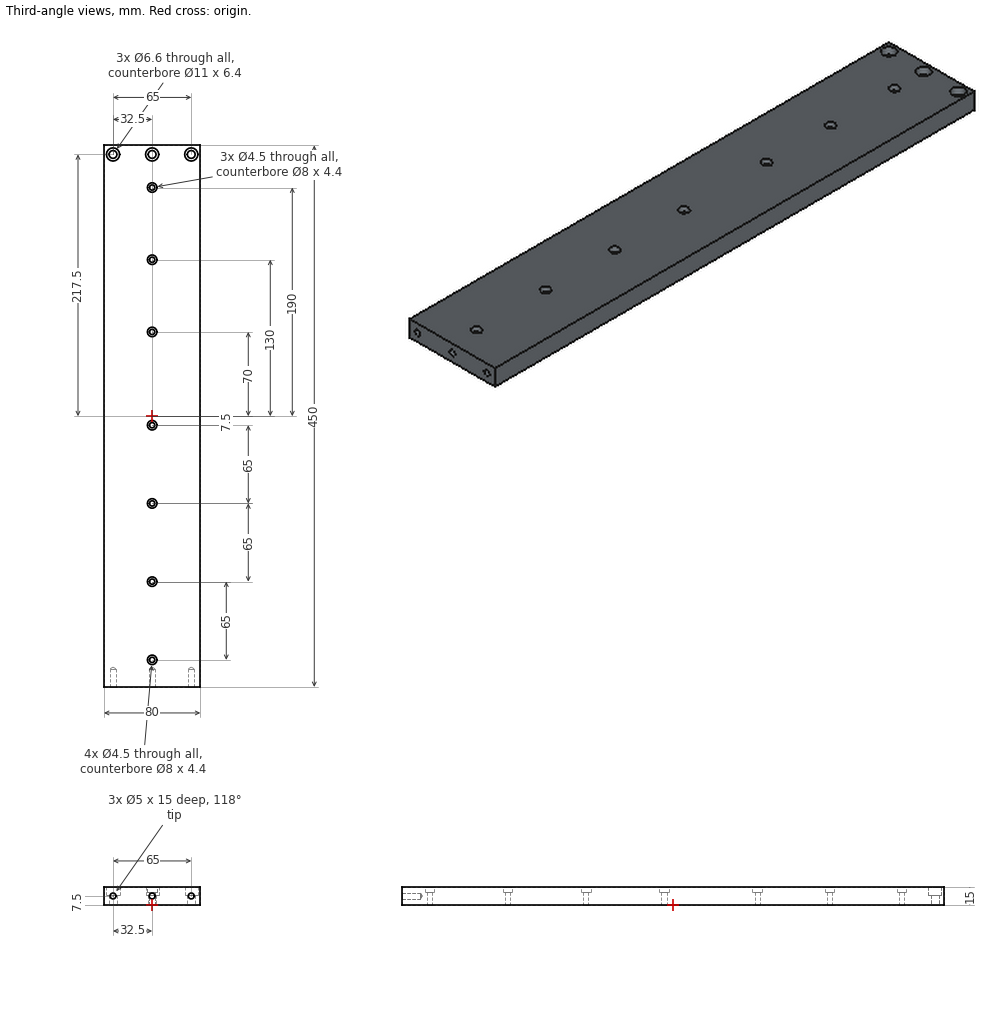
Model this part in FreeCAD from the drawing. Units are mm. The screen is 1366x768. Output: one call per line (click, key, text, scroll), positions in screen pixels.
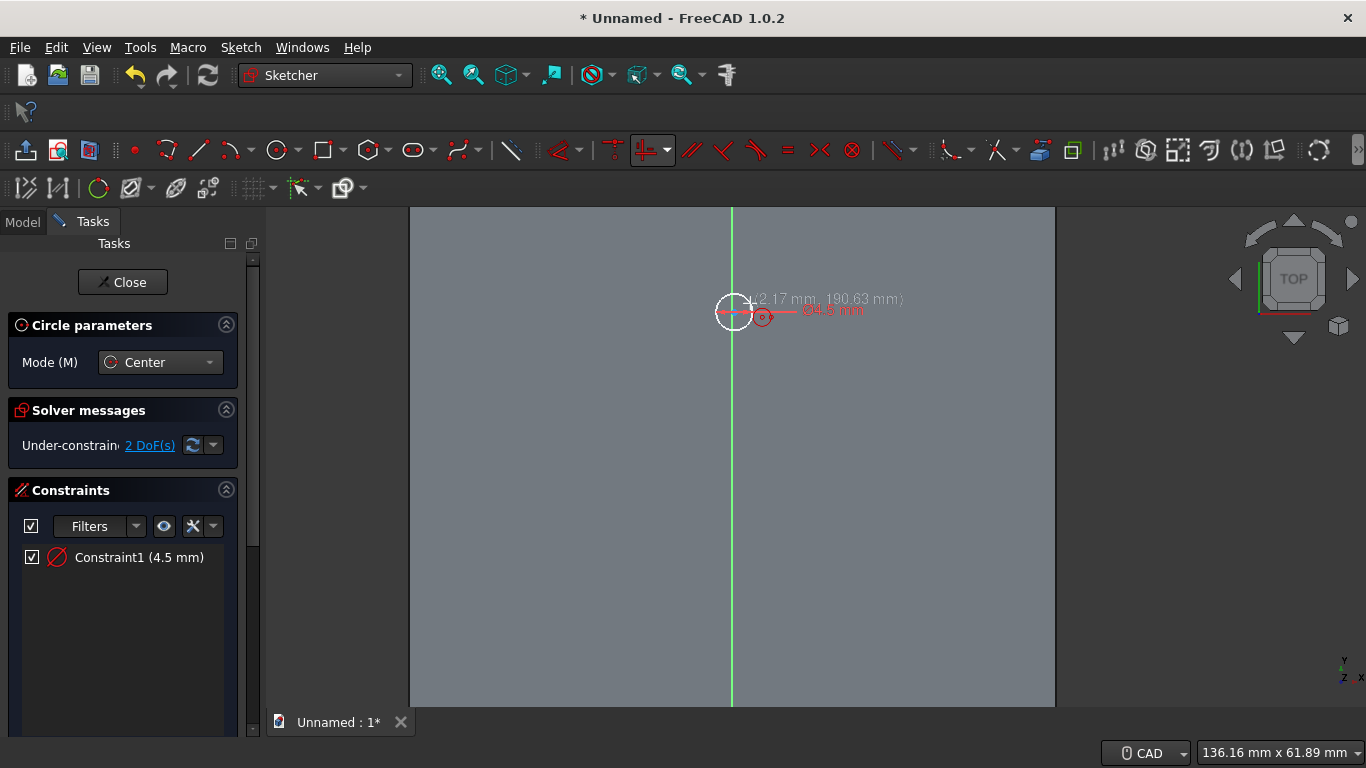
scroll(751, 303, down, 8)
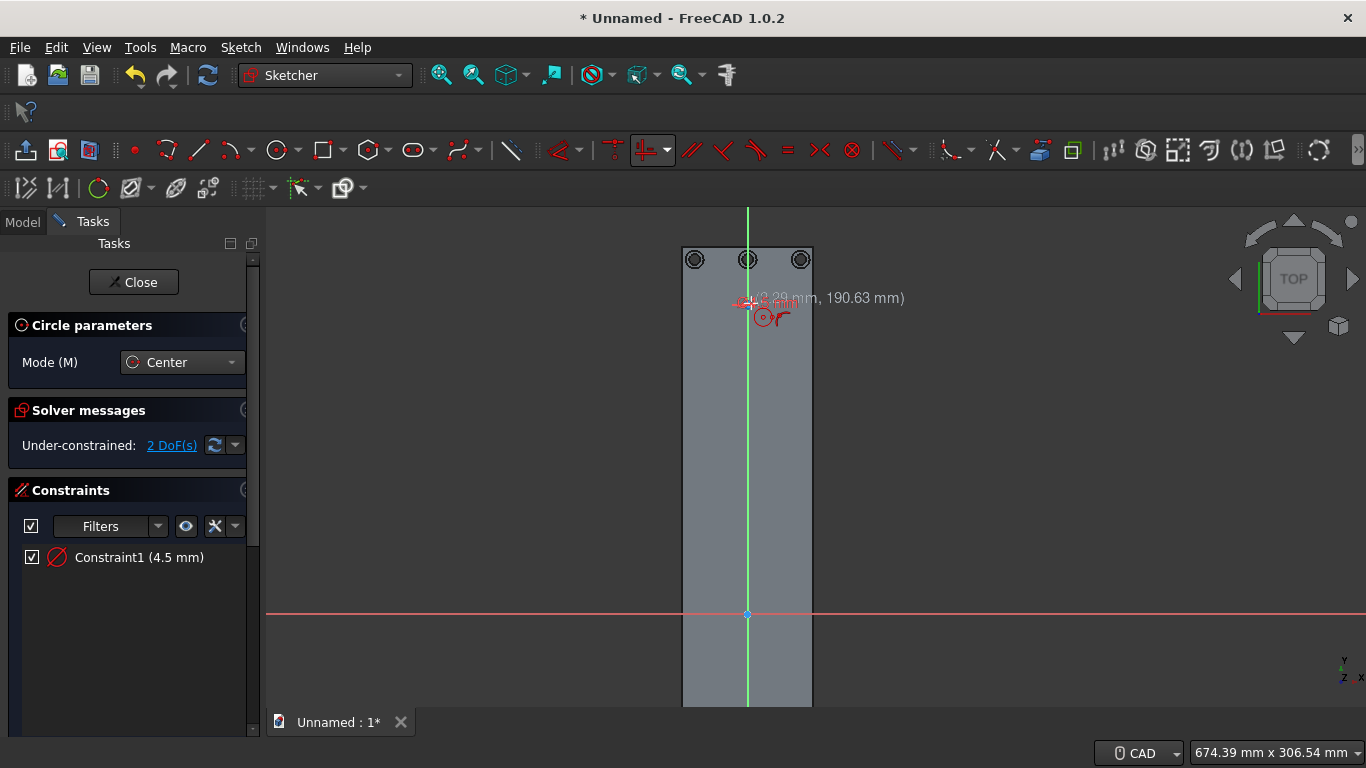
scroll(748, 402, up, 10)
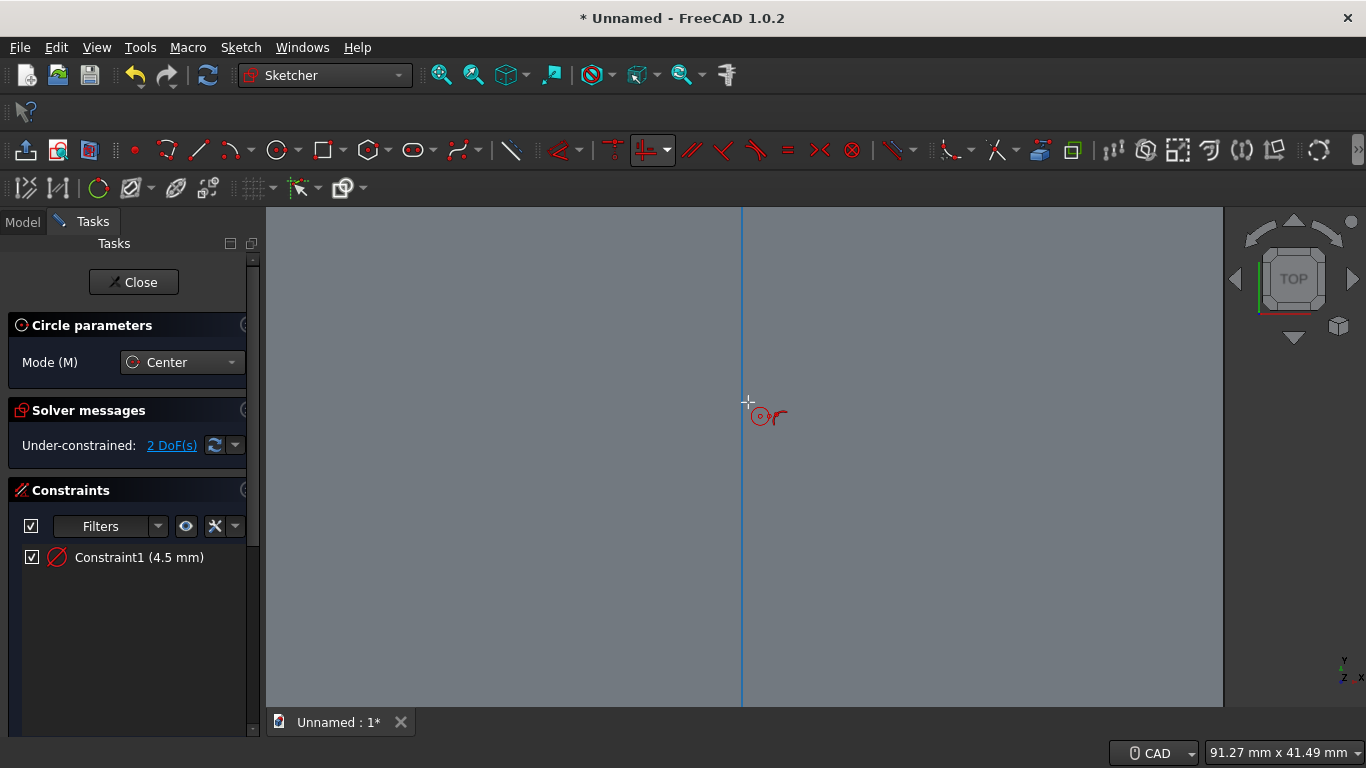
scroll(748, 402, down, 10)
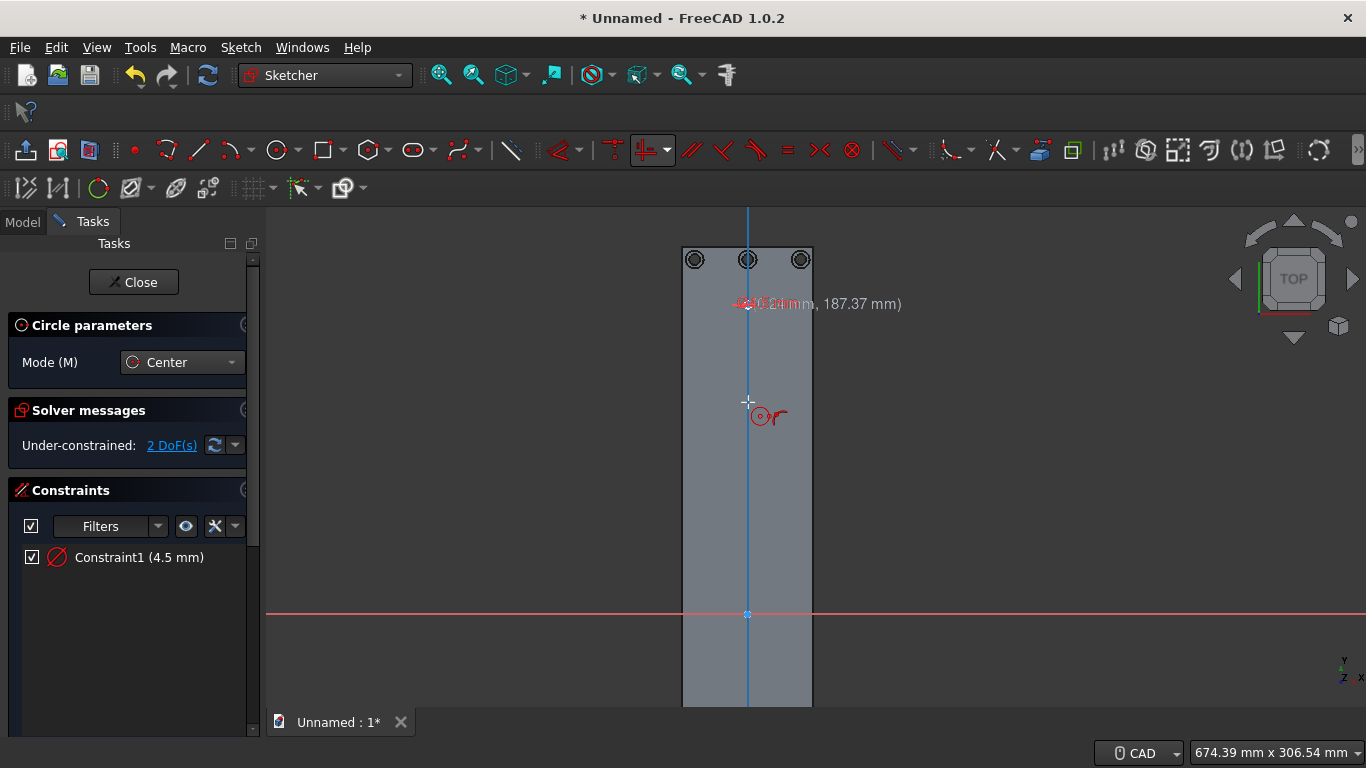
click(748, 402)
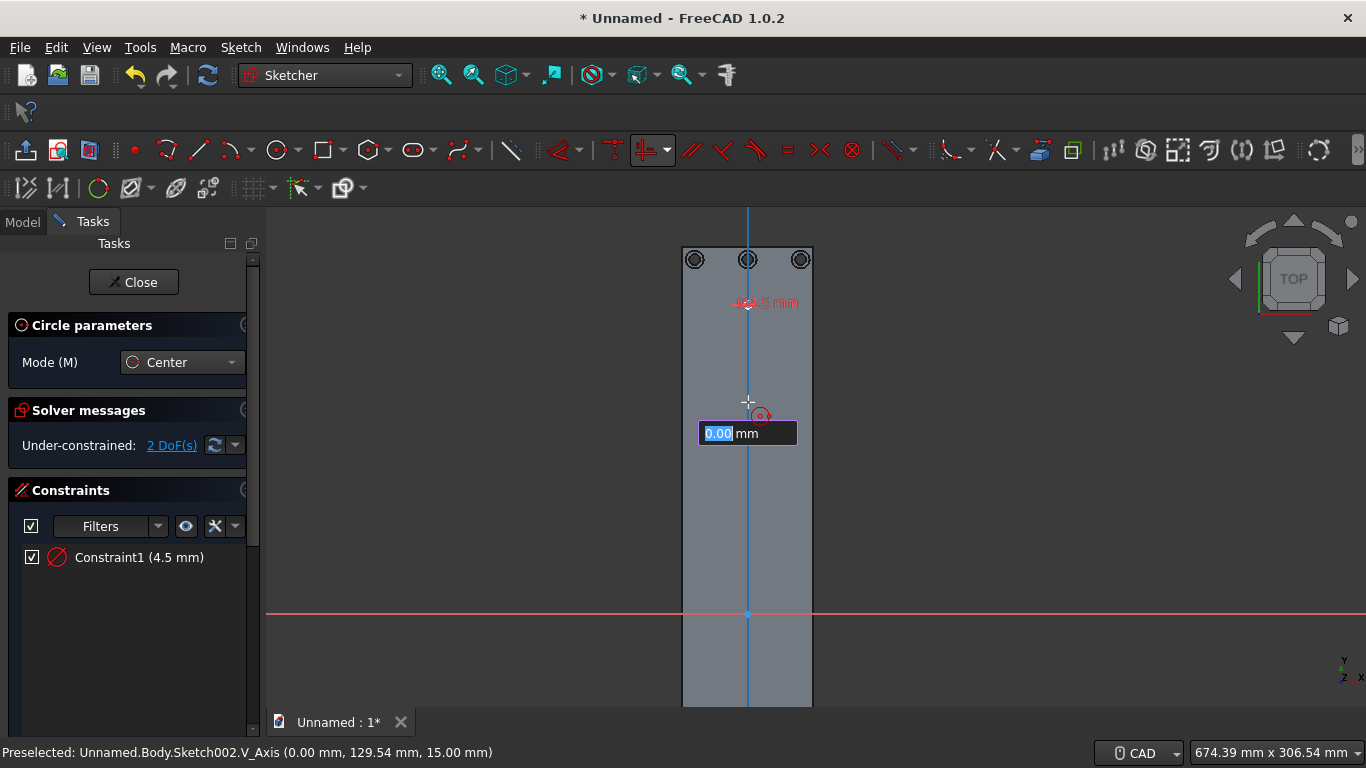
scroll(751, 401, up, 8)
move(750, 399)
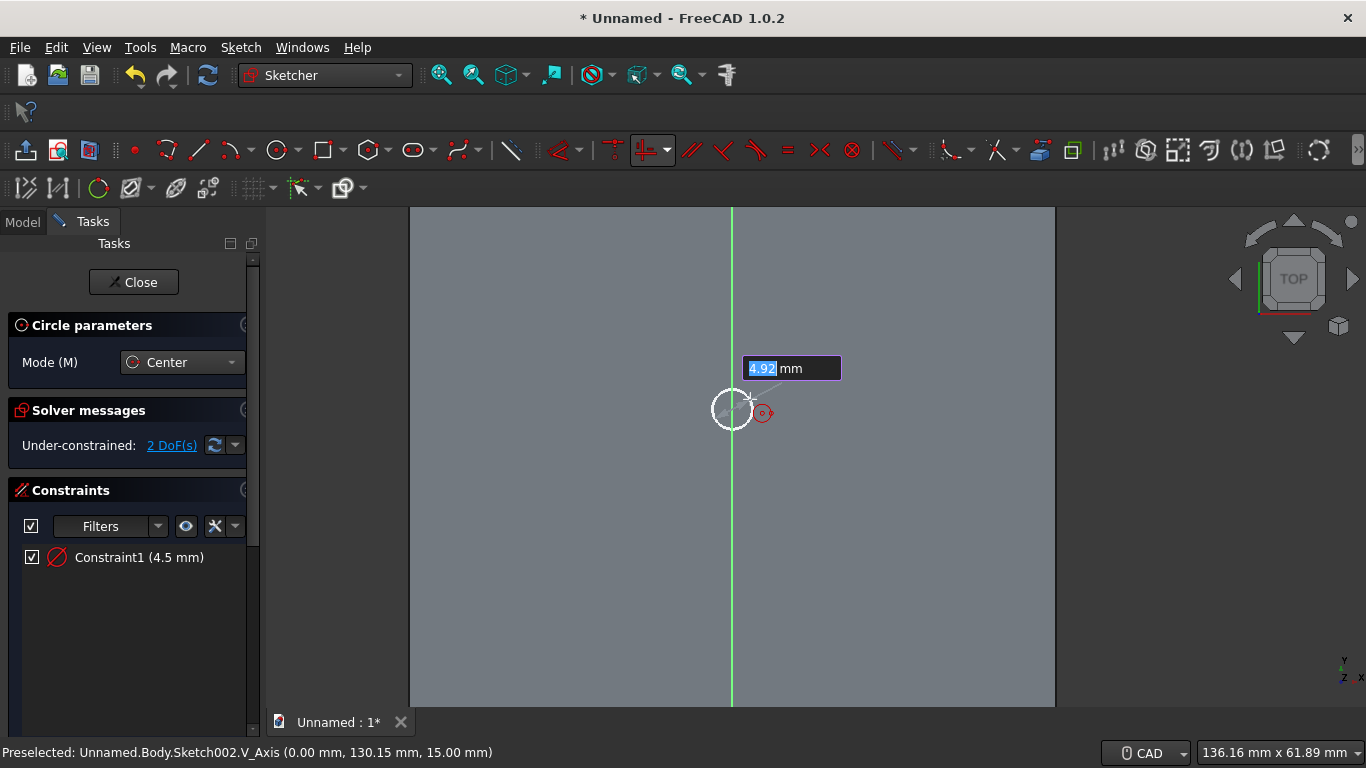
text(4.5)
key(Return)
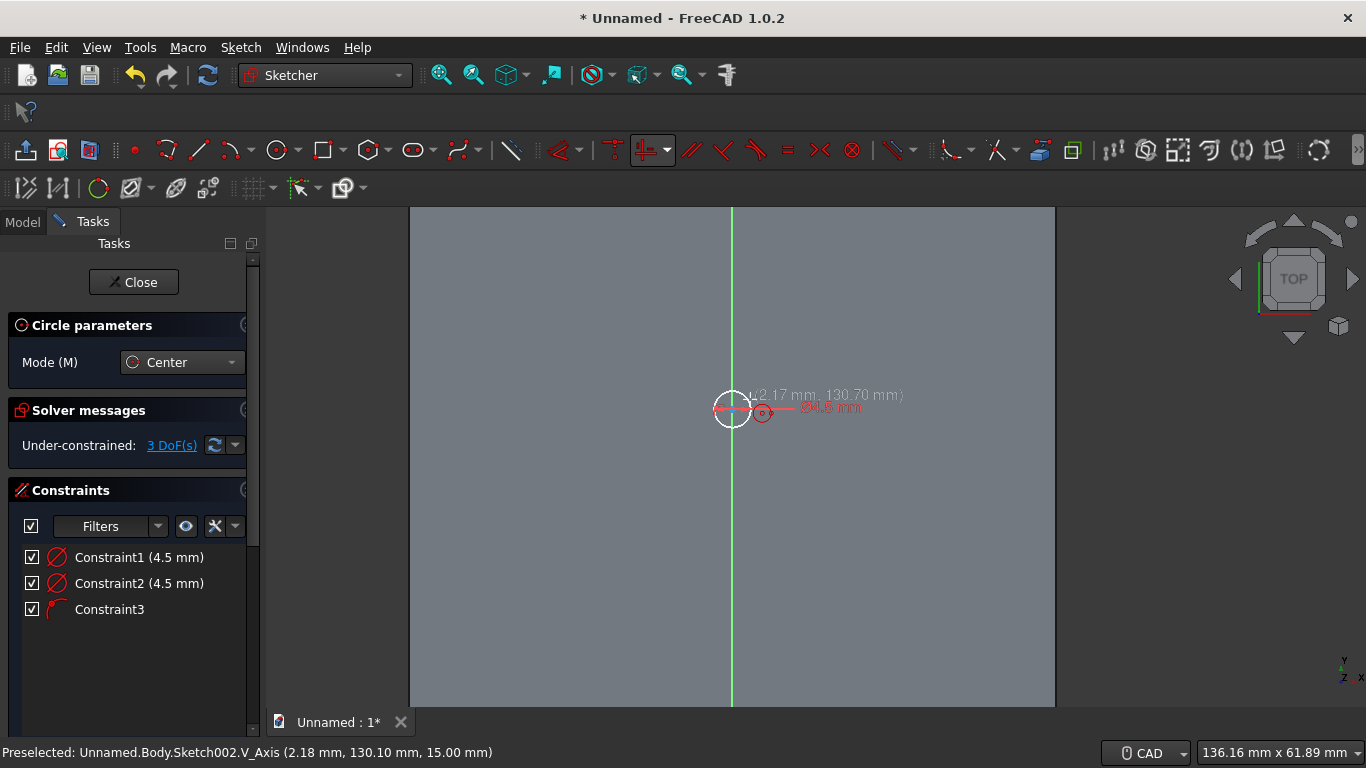
scroll(751, 401, down, 8)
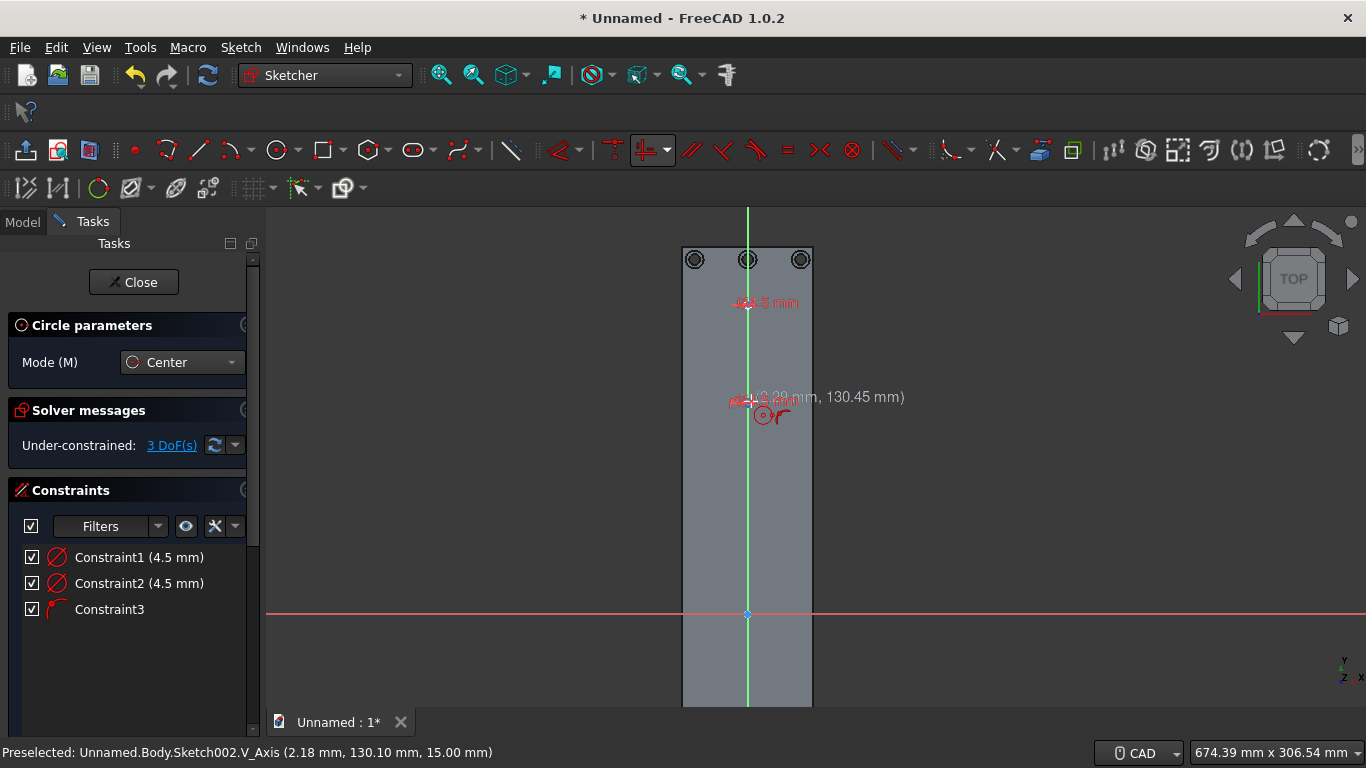
scroll(748, 500, up, 10)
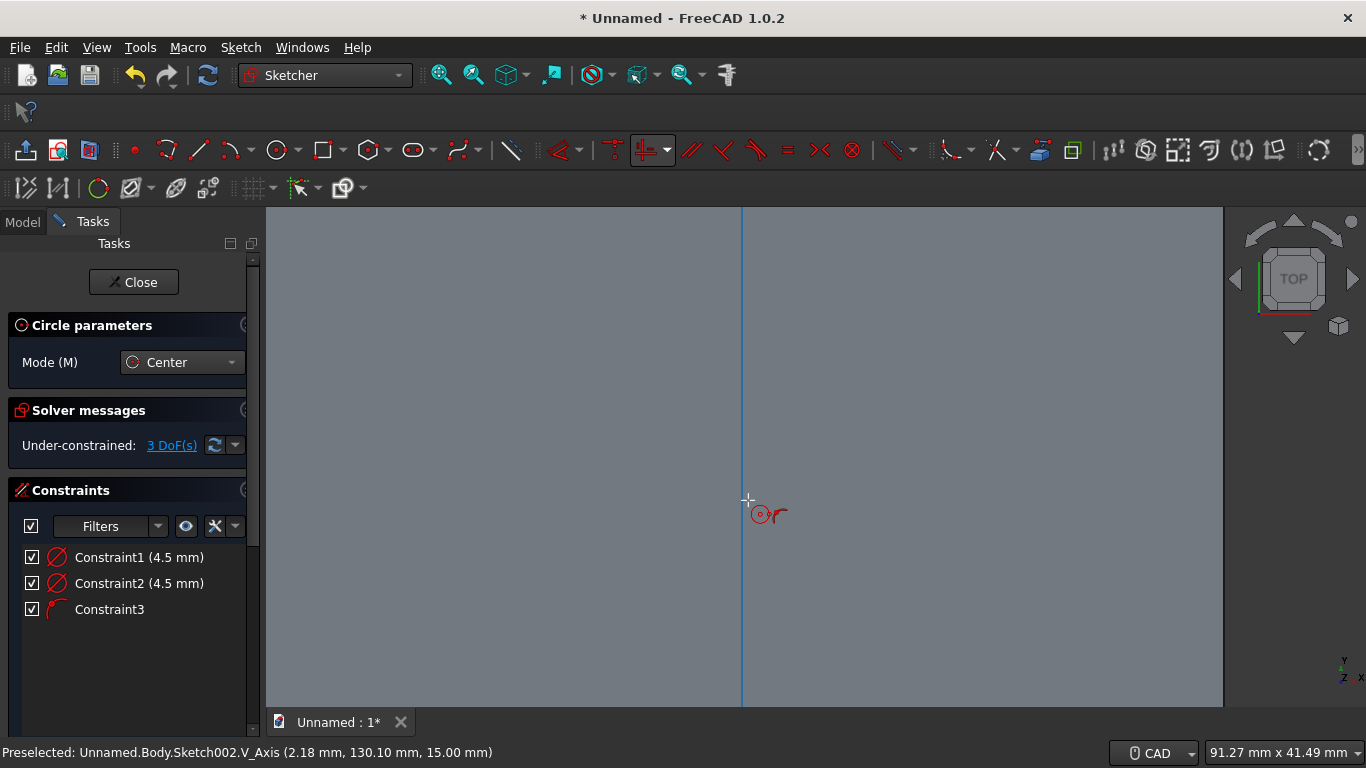
scroll(748, 500, down, 10)